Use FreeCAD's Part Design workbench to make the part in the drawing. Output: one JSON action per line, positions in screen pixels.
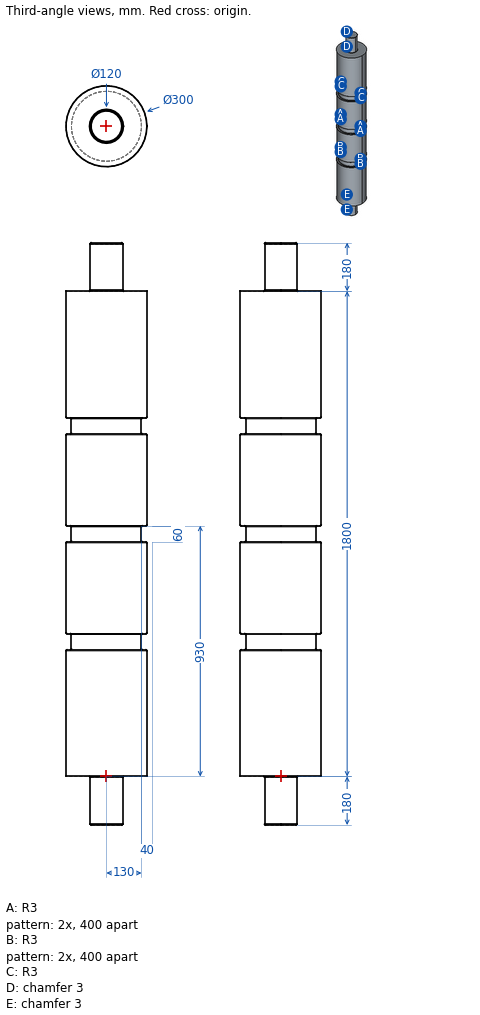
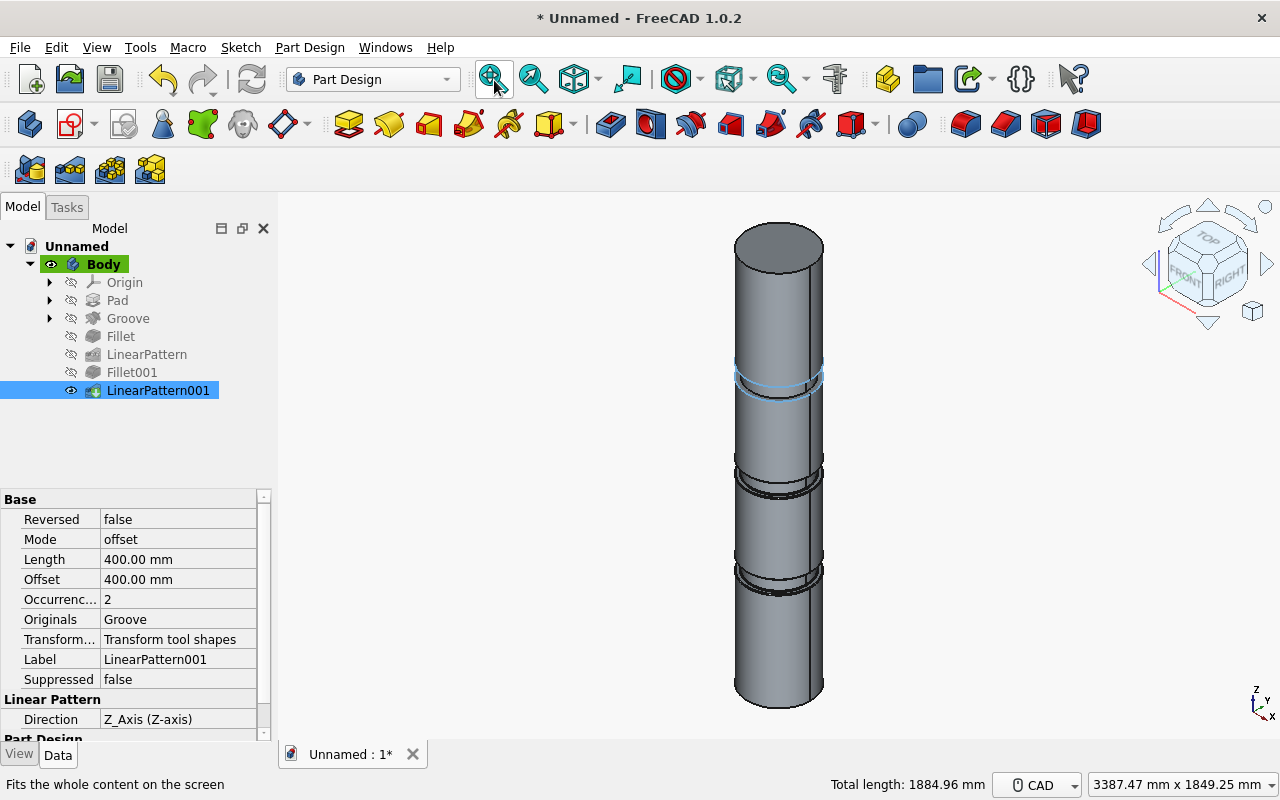
{"action": "key", "text": "1"}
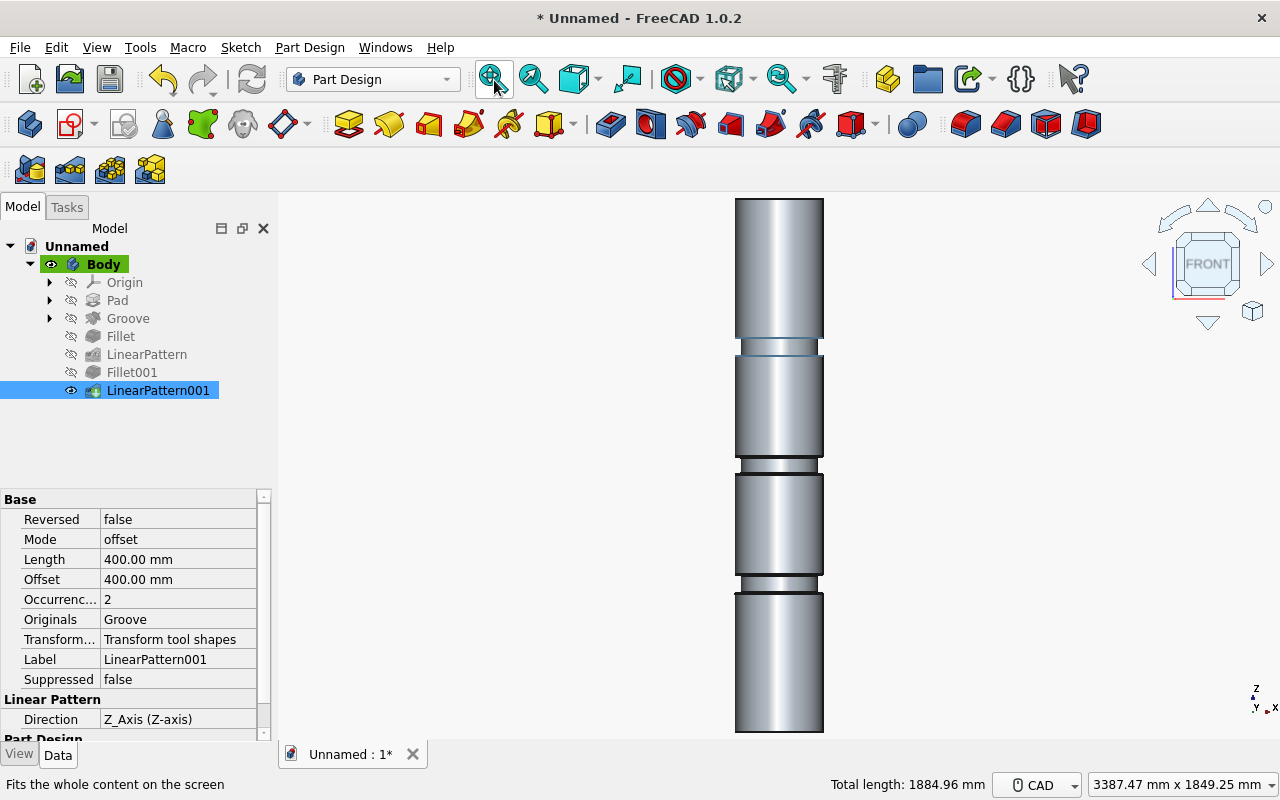
{"action": "key", "text": "3"}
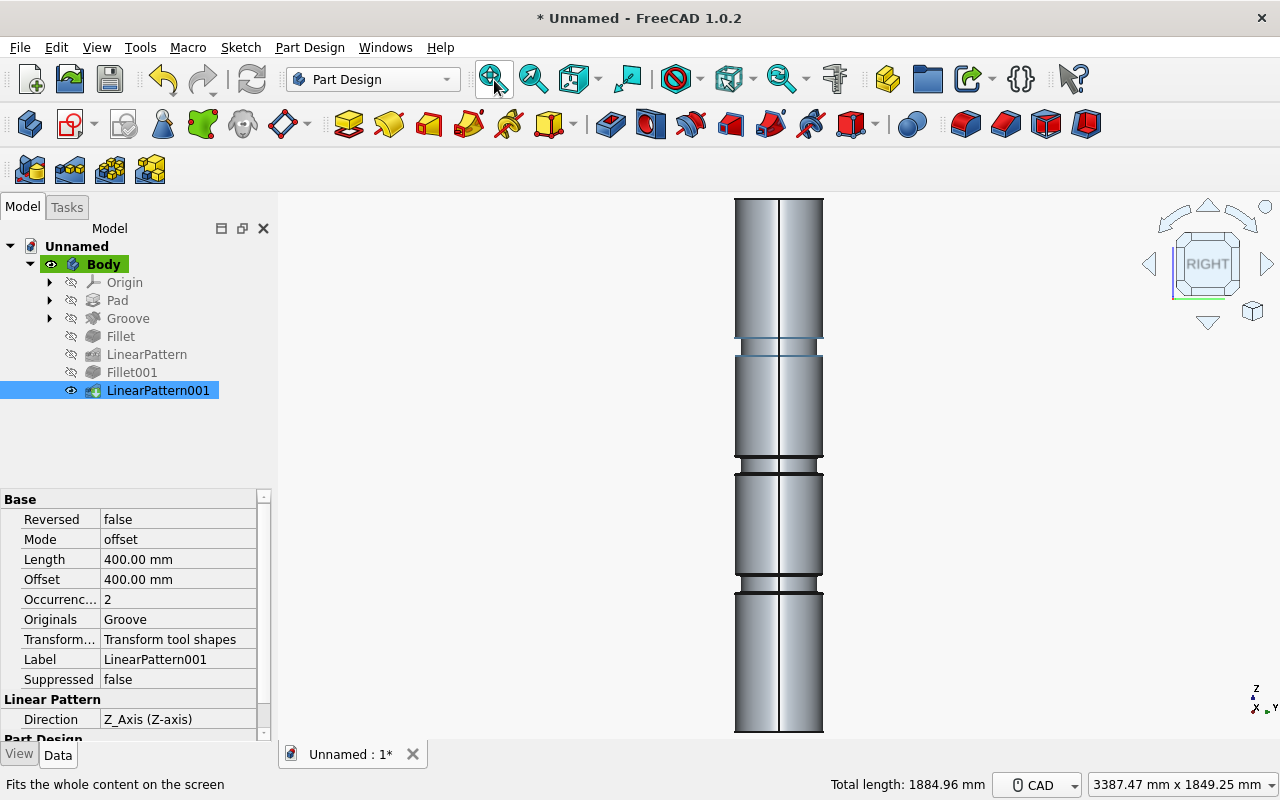
{"action": "key", "text": "5"}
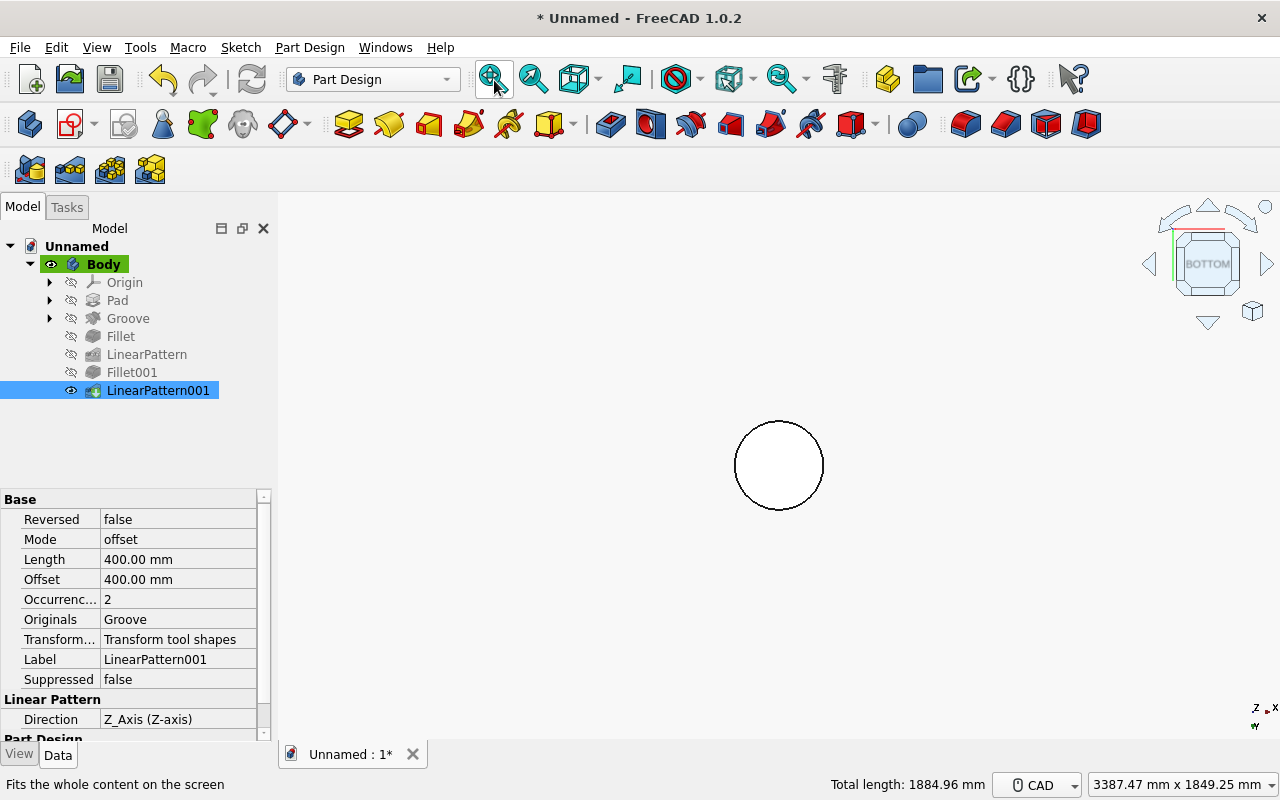
{"action": "left_click", "coordinate": [494, 80]}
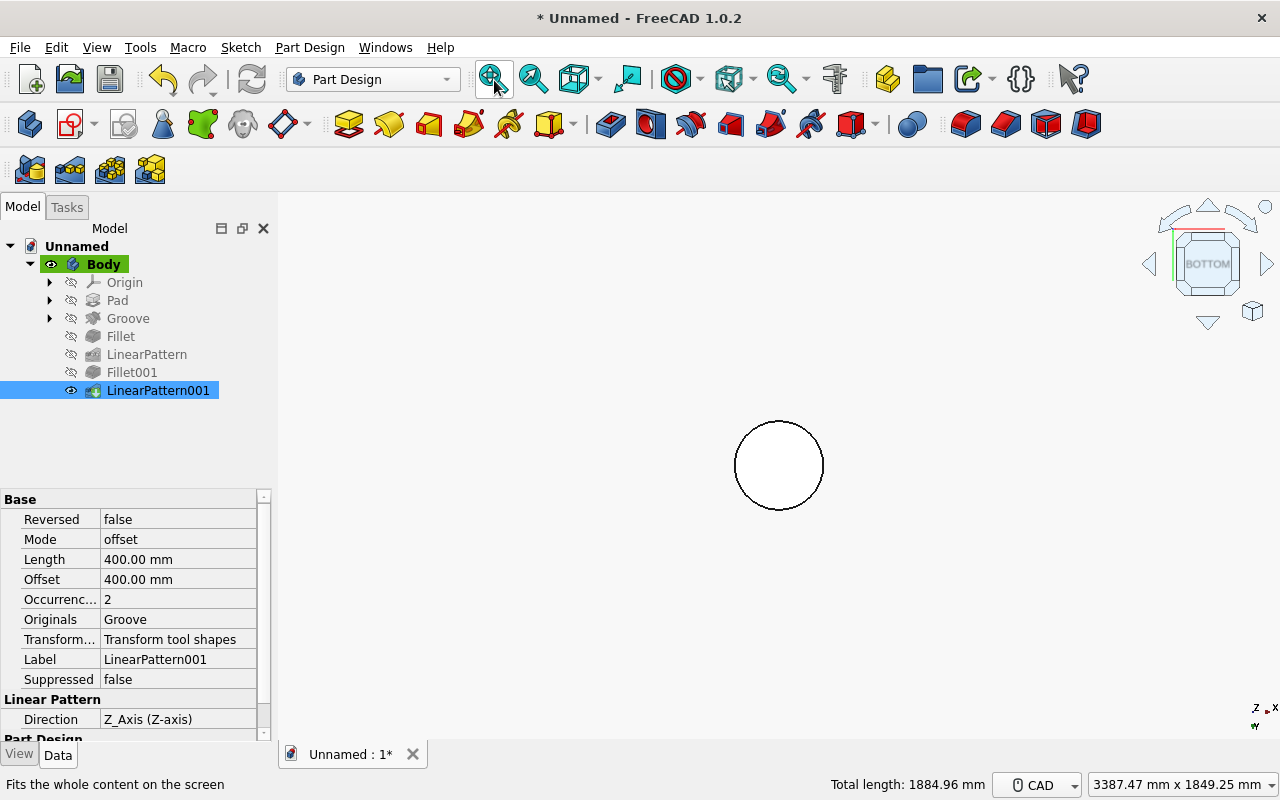
{"action": "key", "text": "4"}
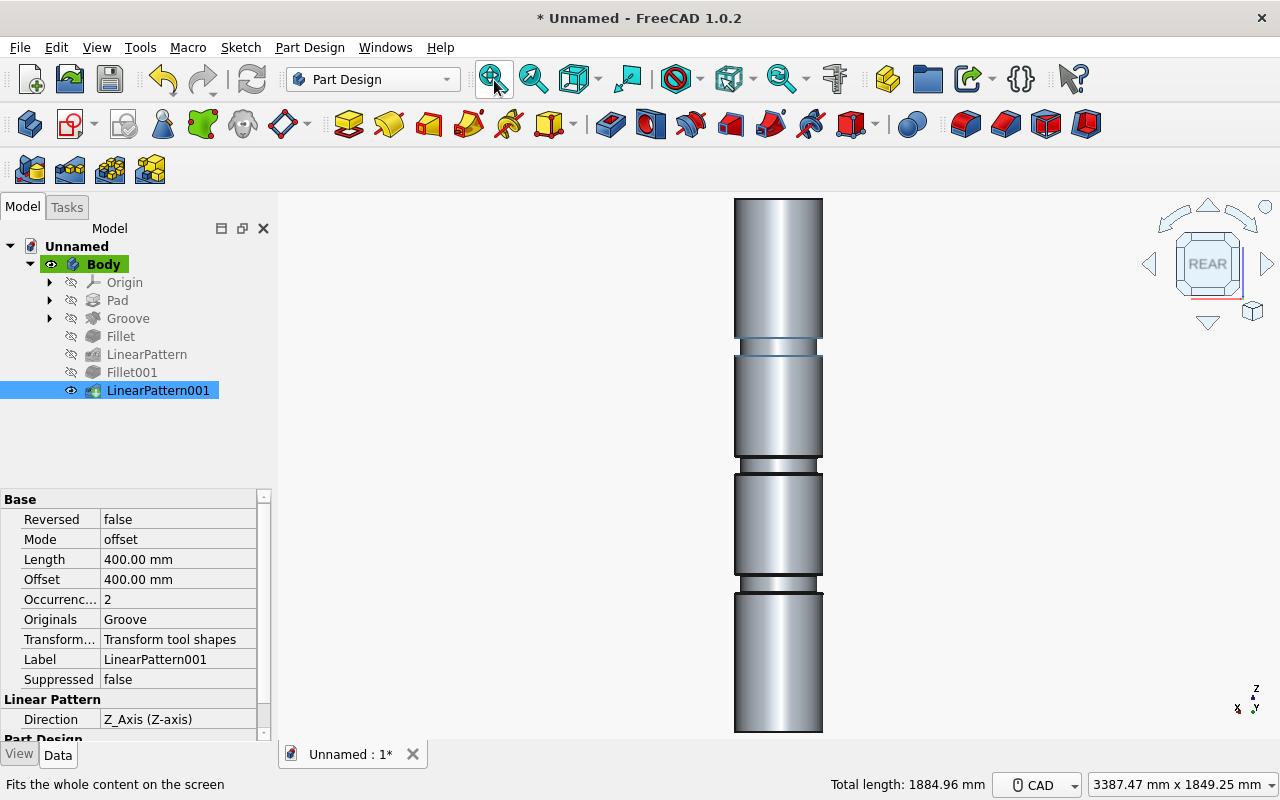
{"action": "key", "text": "6"}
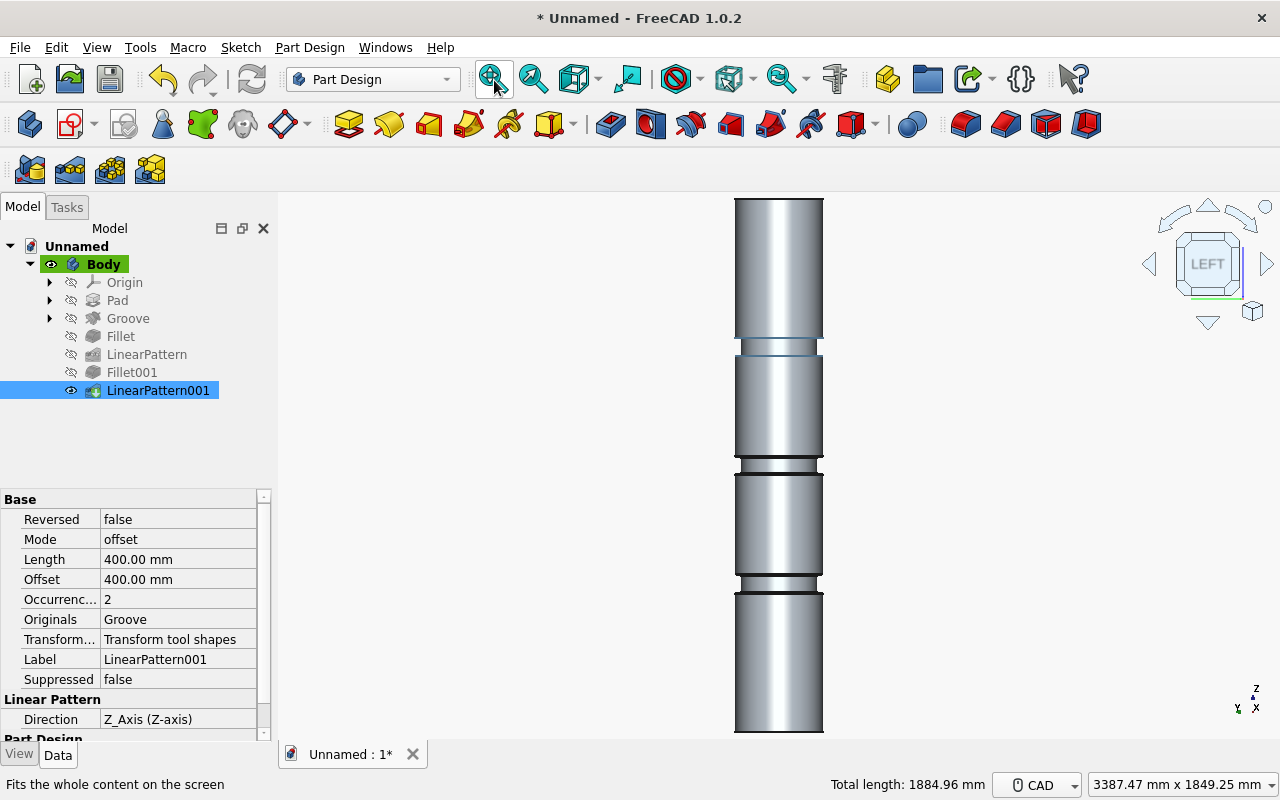
{"action": "key", "text": "v 3"}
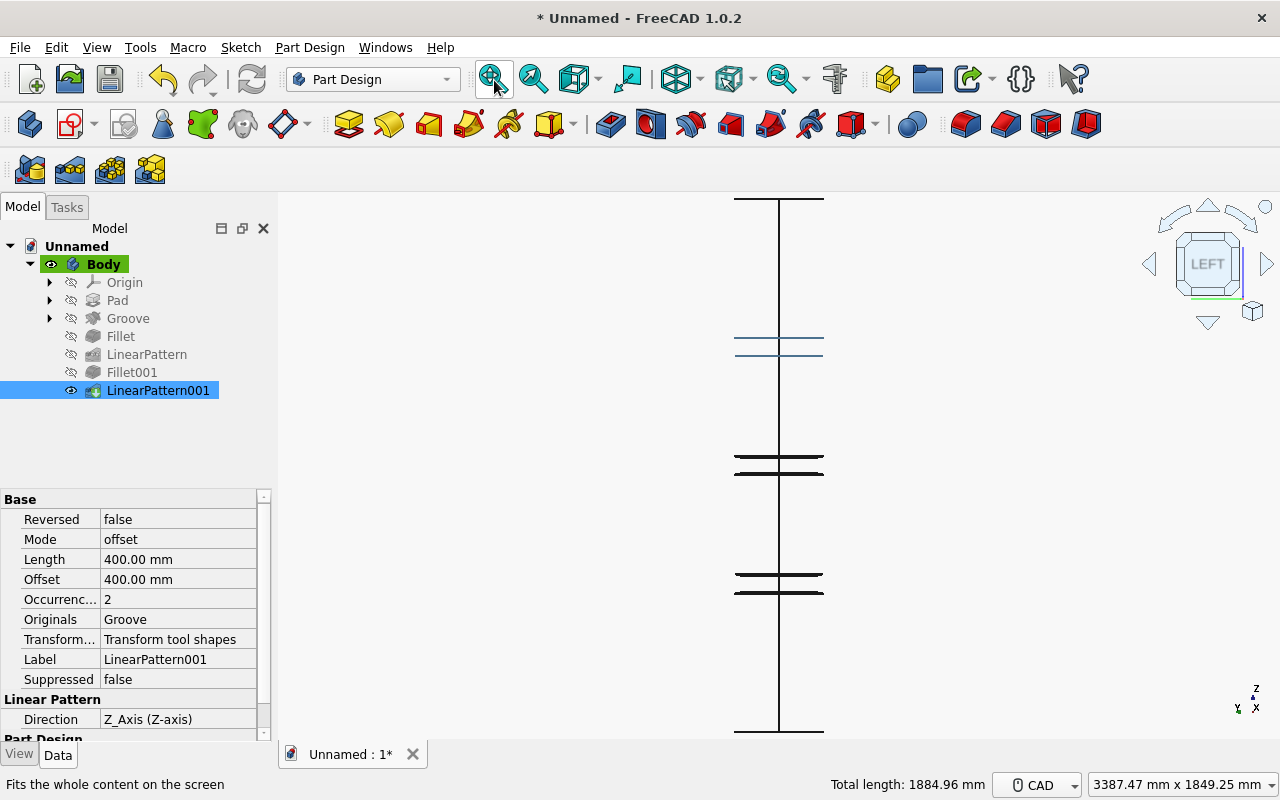
{"action": "key", "text": "0"}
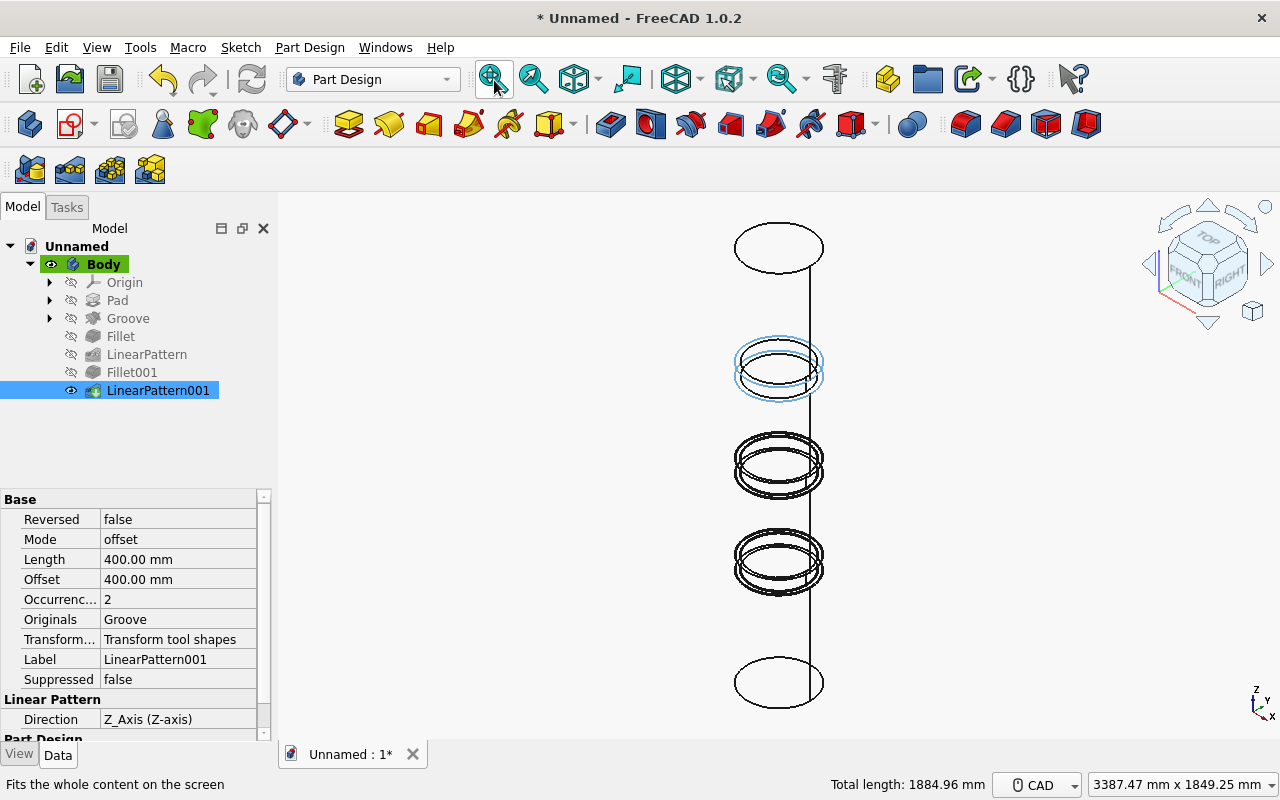
{"action": "left_click", "coordinate": [752, 345], "text": "ctrl"}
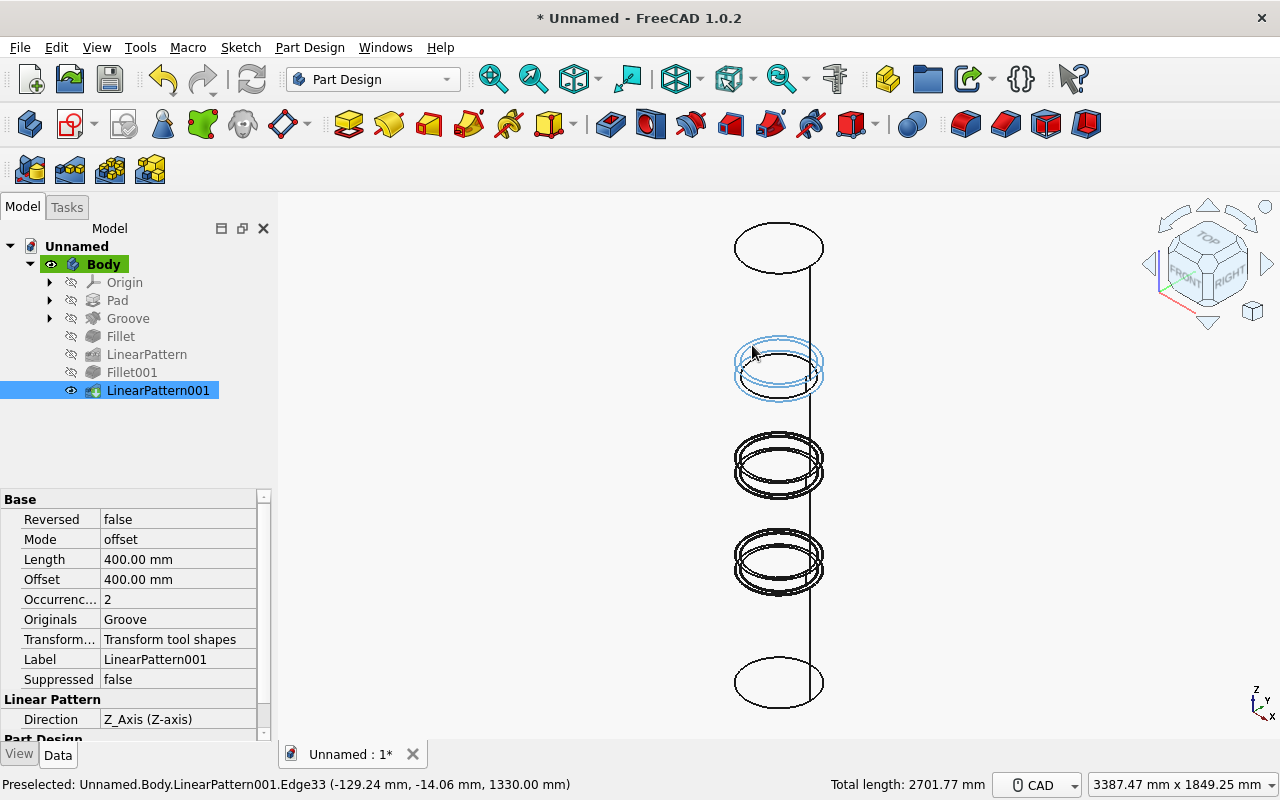
{"action": "left_click", "coordinate": [752, 359], "text": "ctrl"}